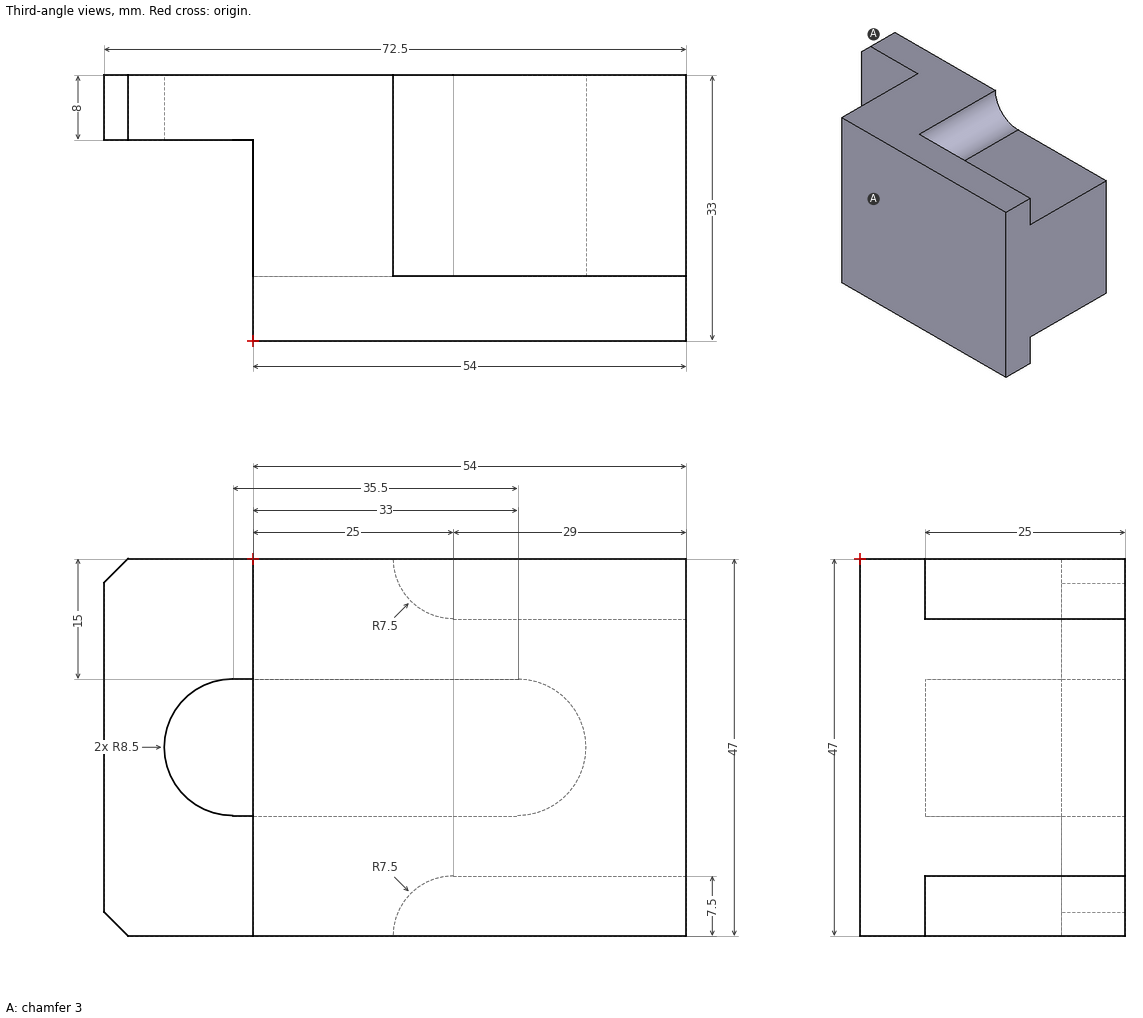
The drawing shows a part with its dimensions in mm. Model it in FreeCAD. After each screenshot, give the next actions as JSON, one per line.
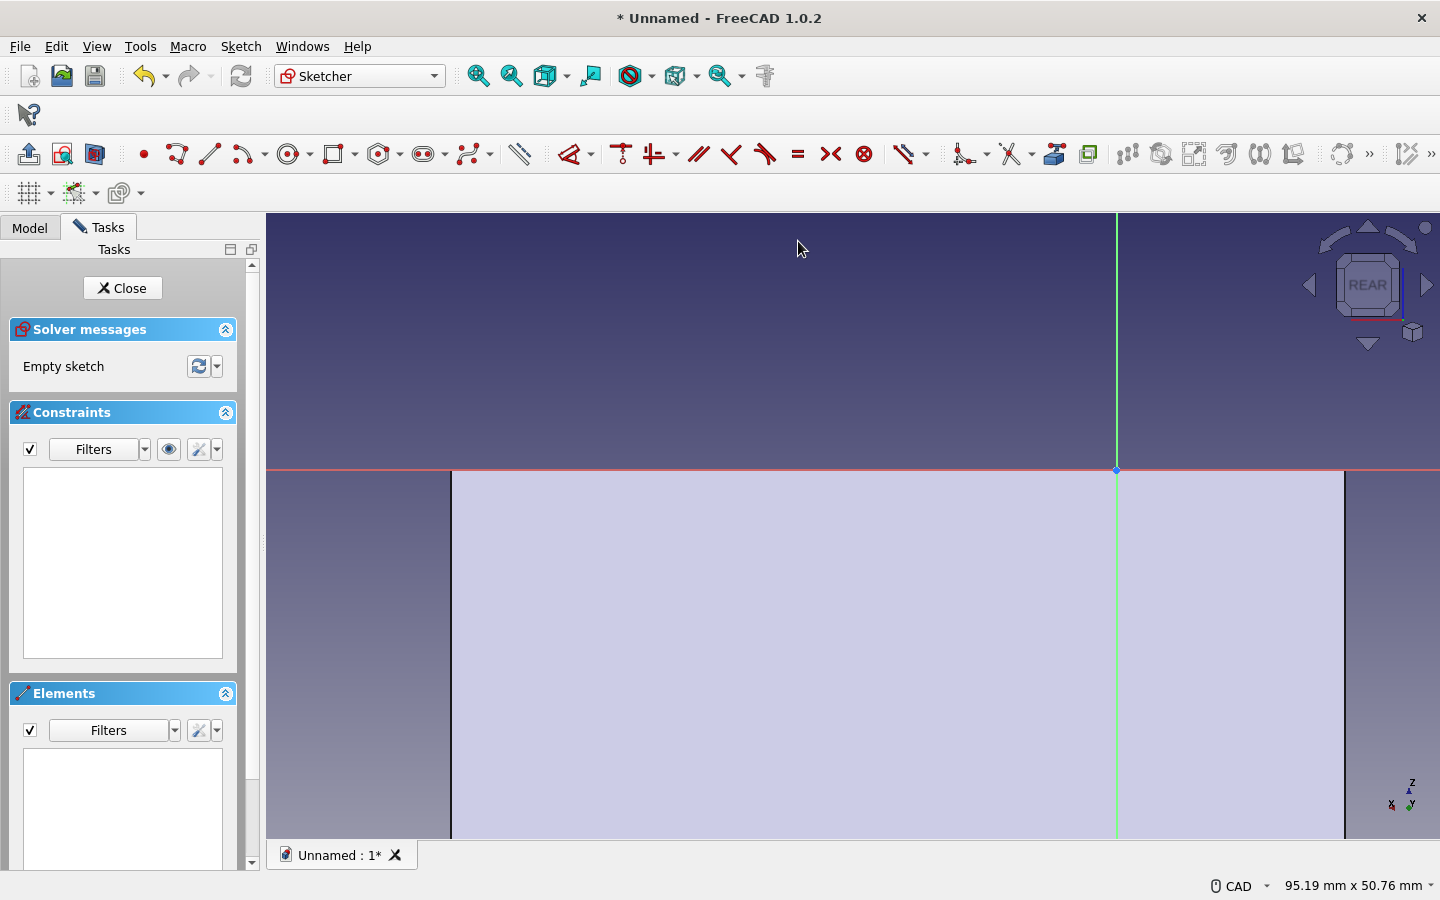
{"action": "key", "text": "g m"}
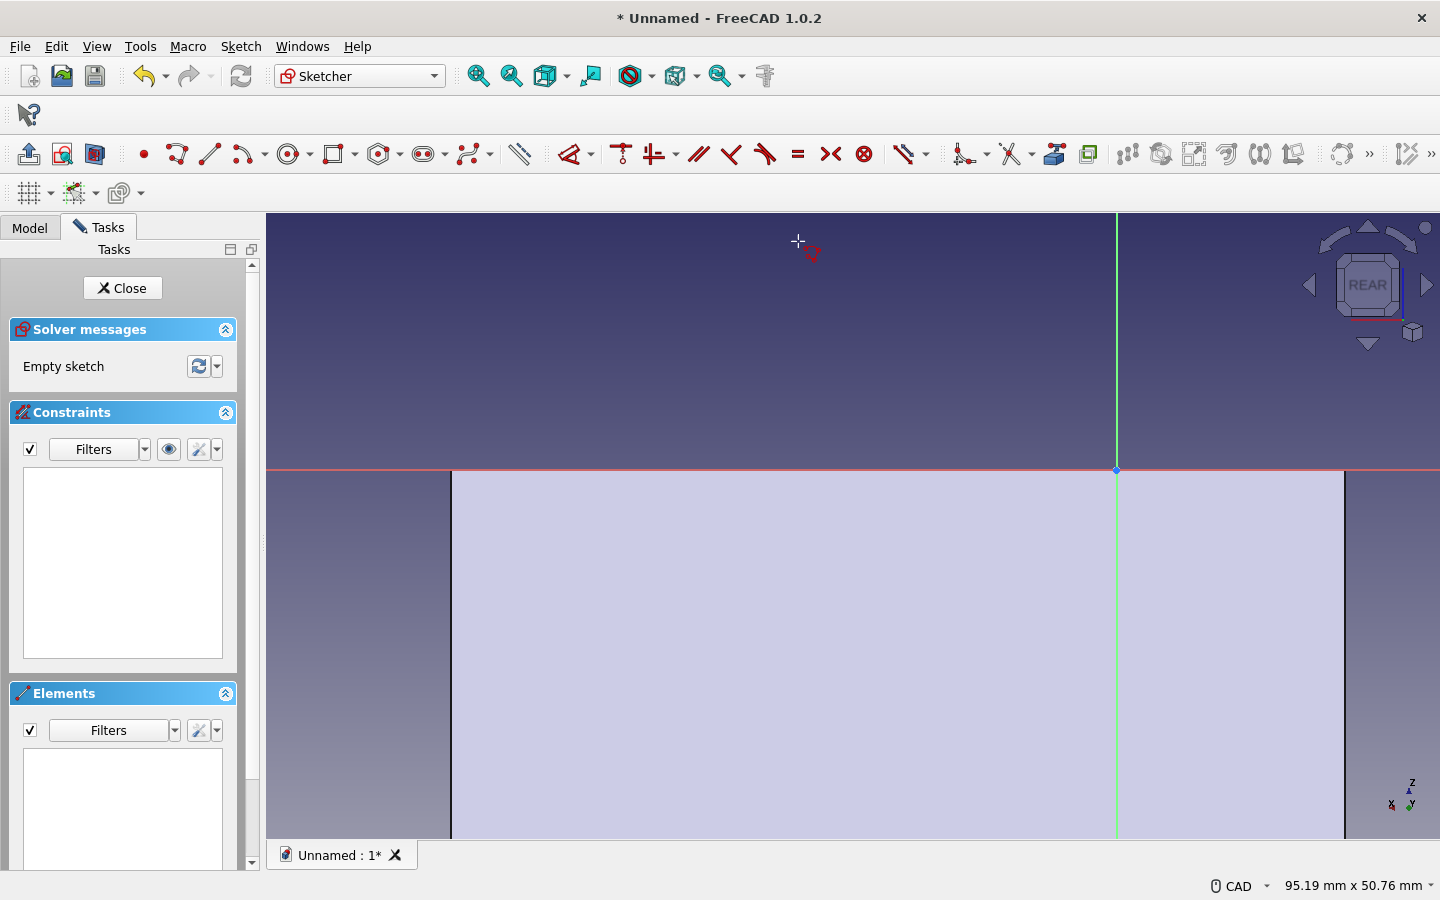
{"action": "left_click", "coordinate": [901, 470]}
{"action": "left_click", "coordinate": [451, 479]}
{"action": "left_click", "coordinate": [451, 563]}
{"action": "left_click", "coordinate": [808, 563]}
{"action": "right_click", "coordinate": [808, 563]}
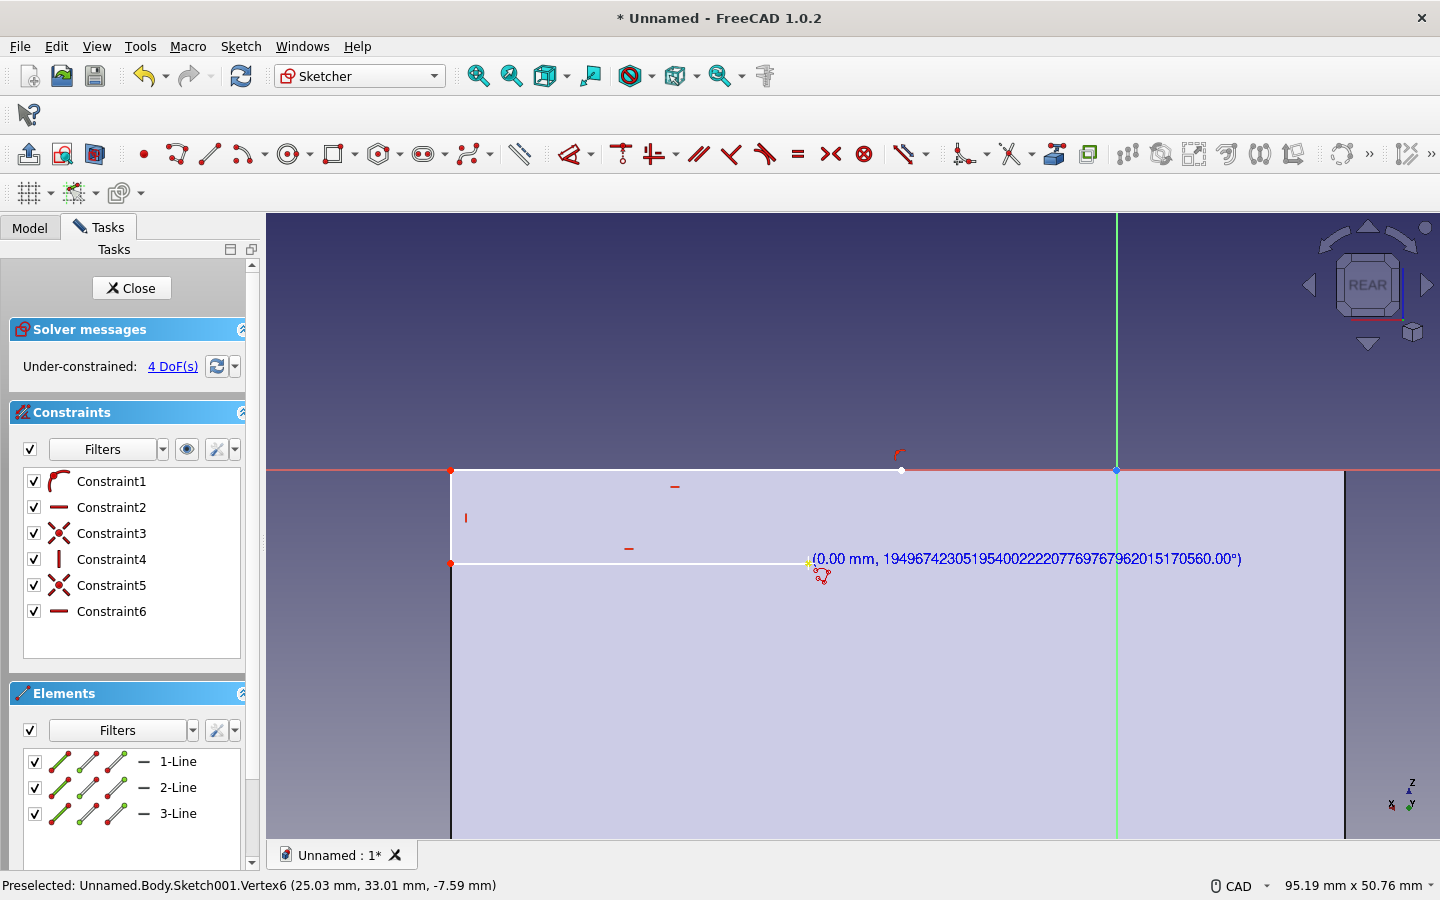
{"action": "key", "text": "g 3 a"}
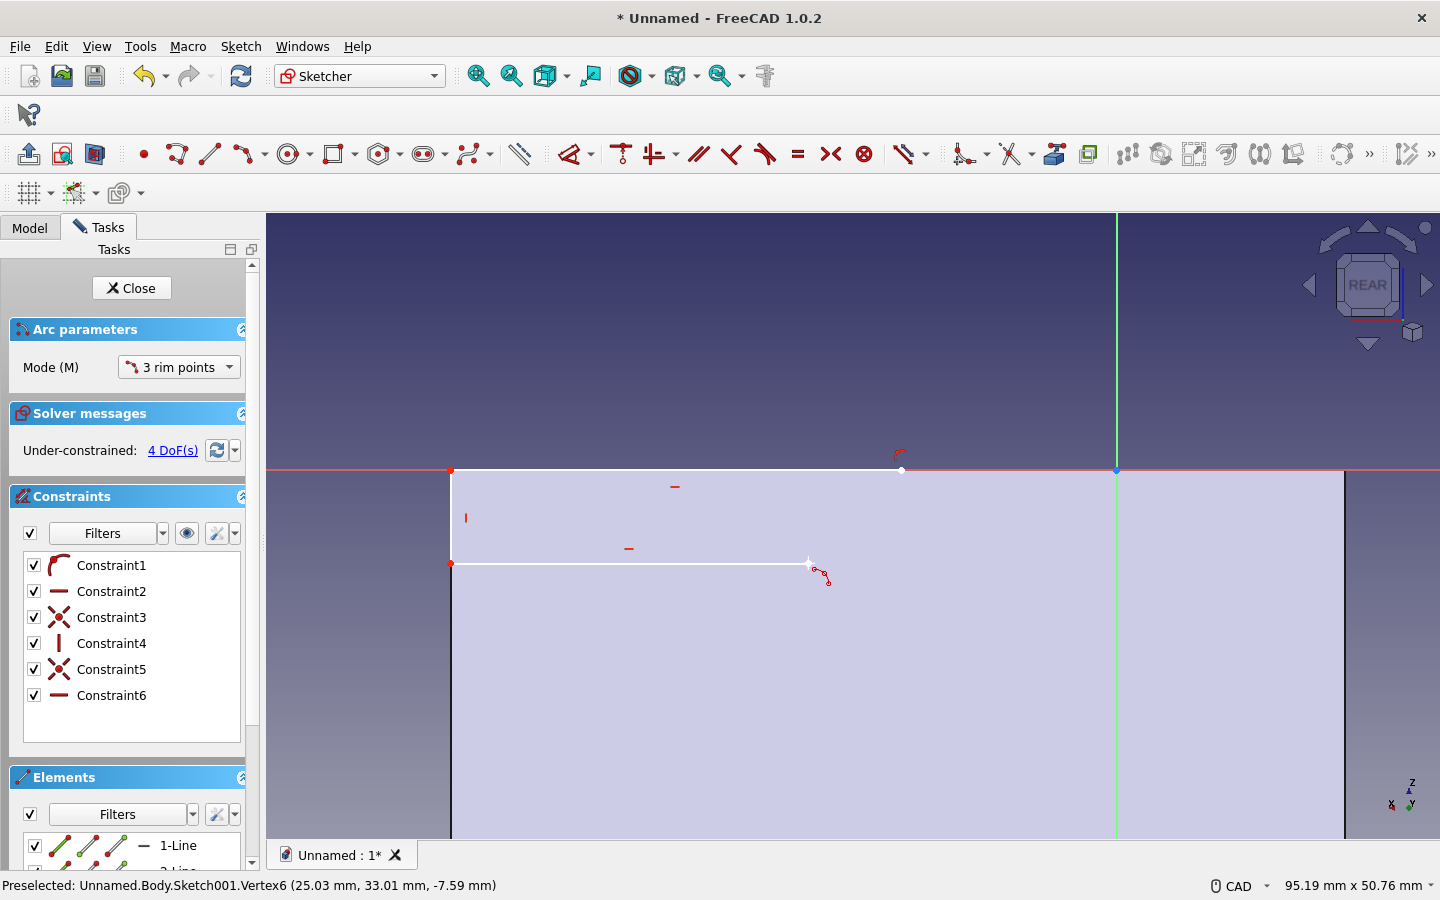
{"action": "left_click", "coordinate": [808, 564]}
{"action": "left_click", "coordinate": [901, 470]}
{"action": "left_click", "coordinate": [874, 536]}
{"action": "key", "text": "Escape"}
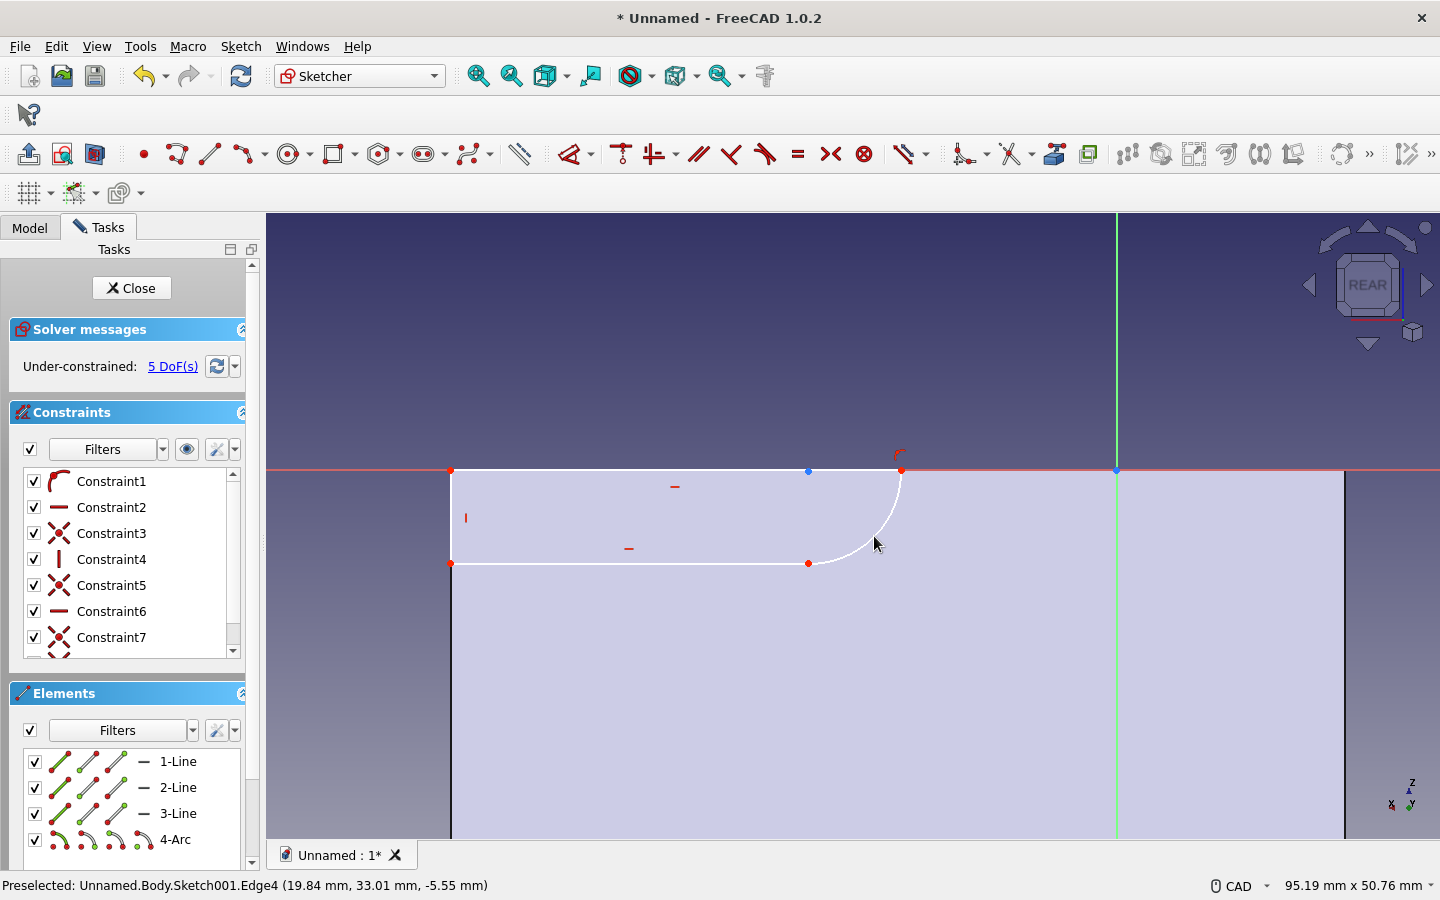
{"action": "left_click", "coordinate": [558, 564]}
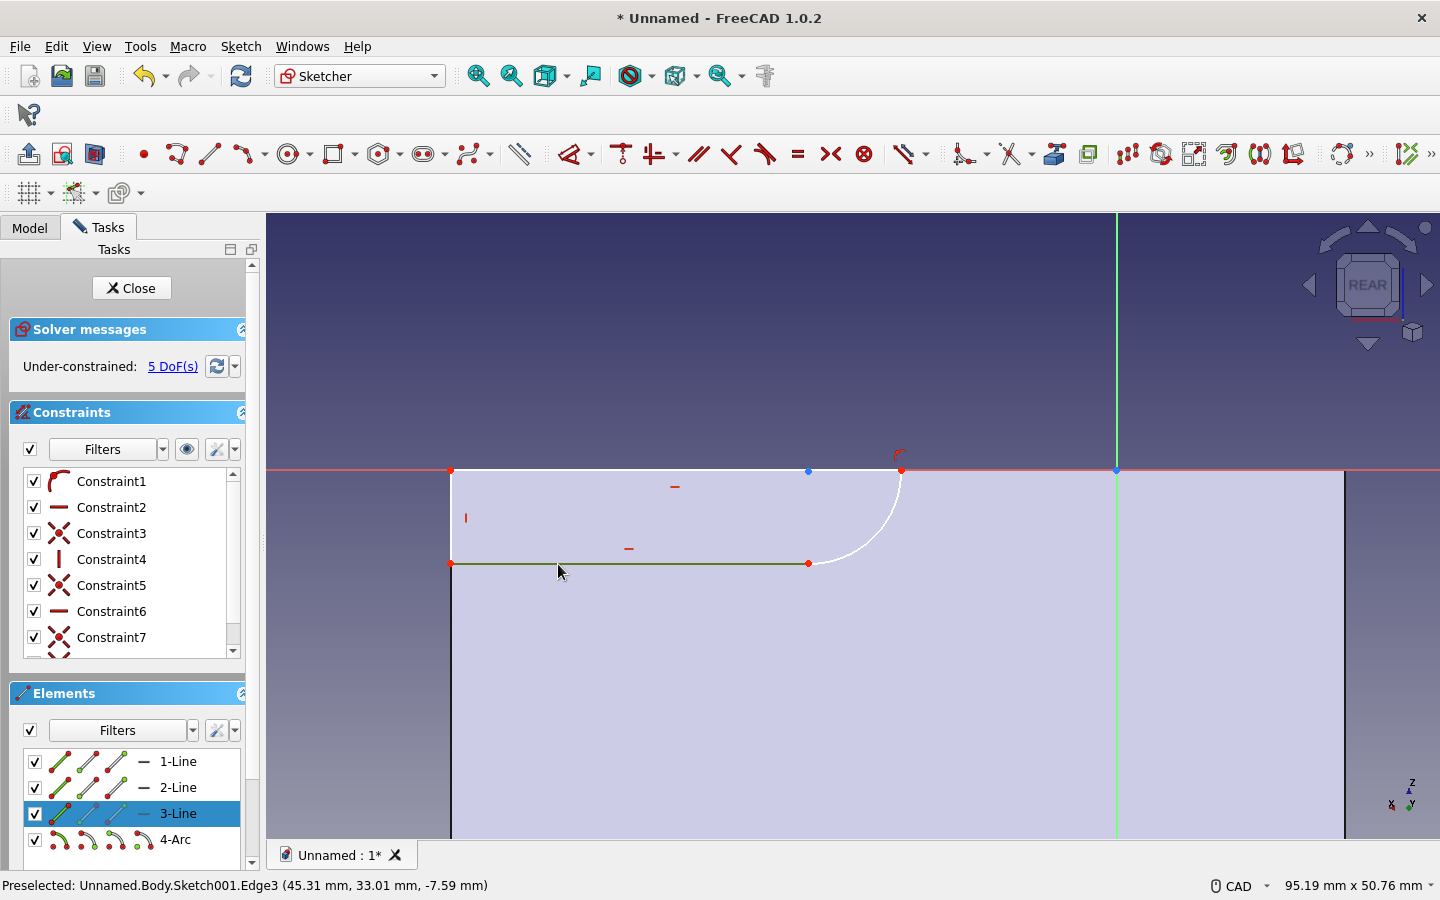
{"action": "left_click", "coordinate": [851, 554]}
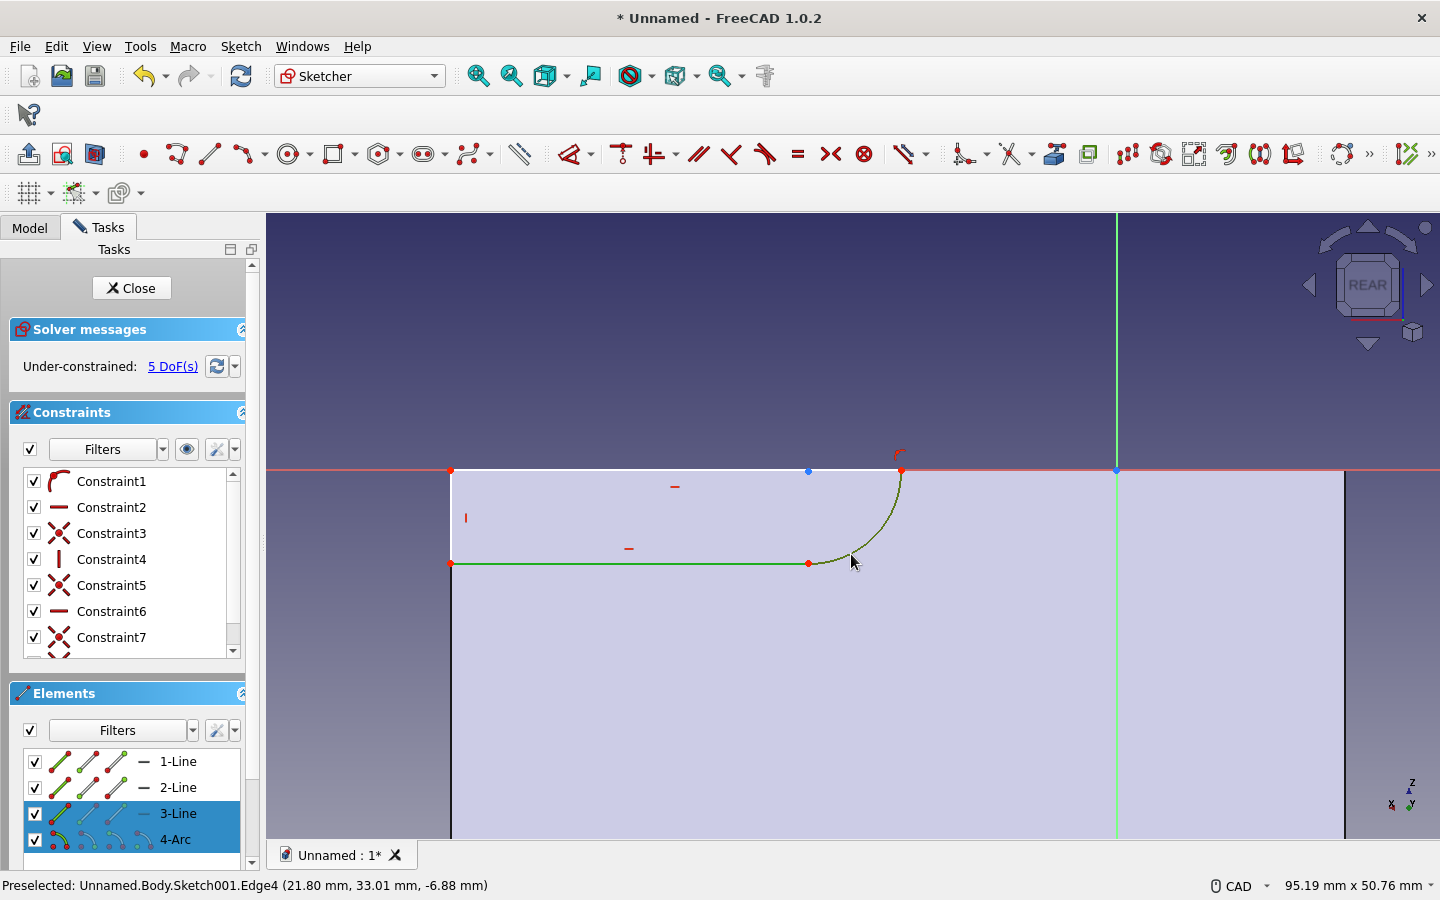
{"action": "left_click", "coordinate": [765, 154]}